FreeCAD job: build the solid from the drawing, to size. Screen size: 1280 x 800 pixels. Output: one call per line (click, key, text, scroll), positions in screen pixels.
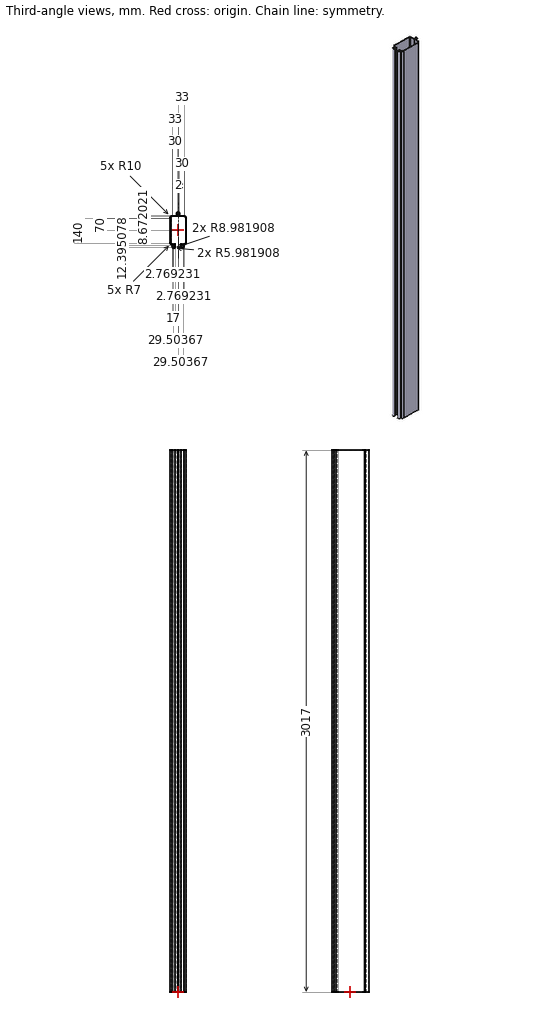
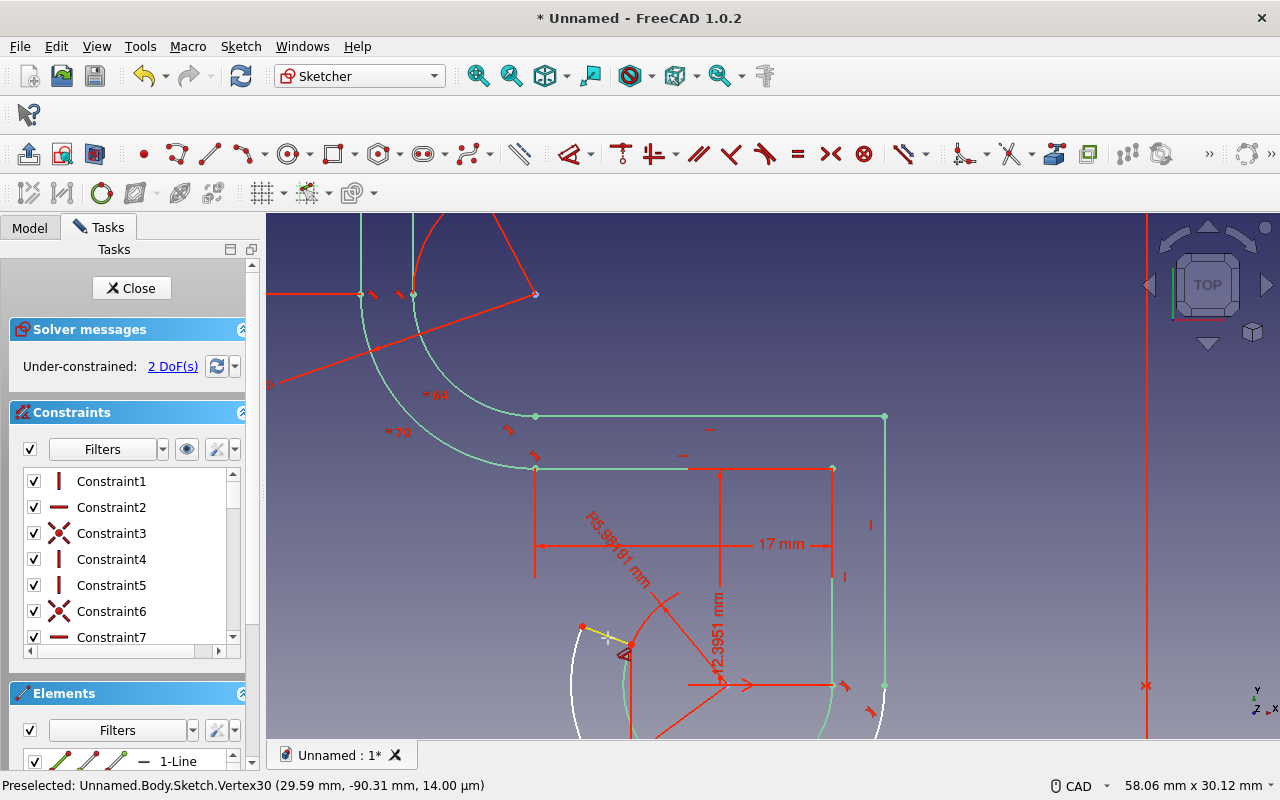
click(607, 636)
click(607, 679)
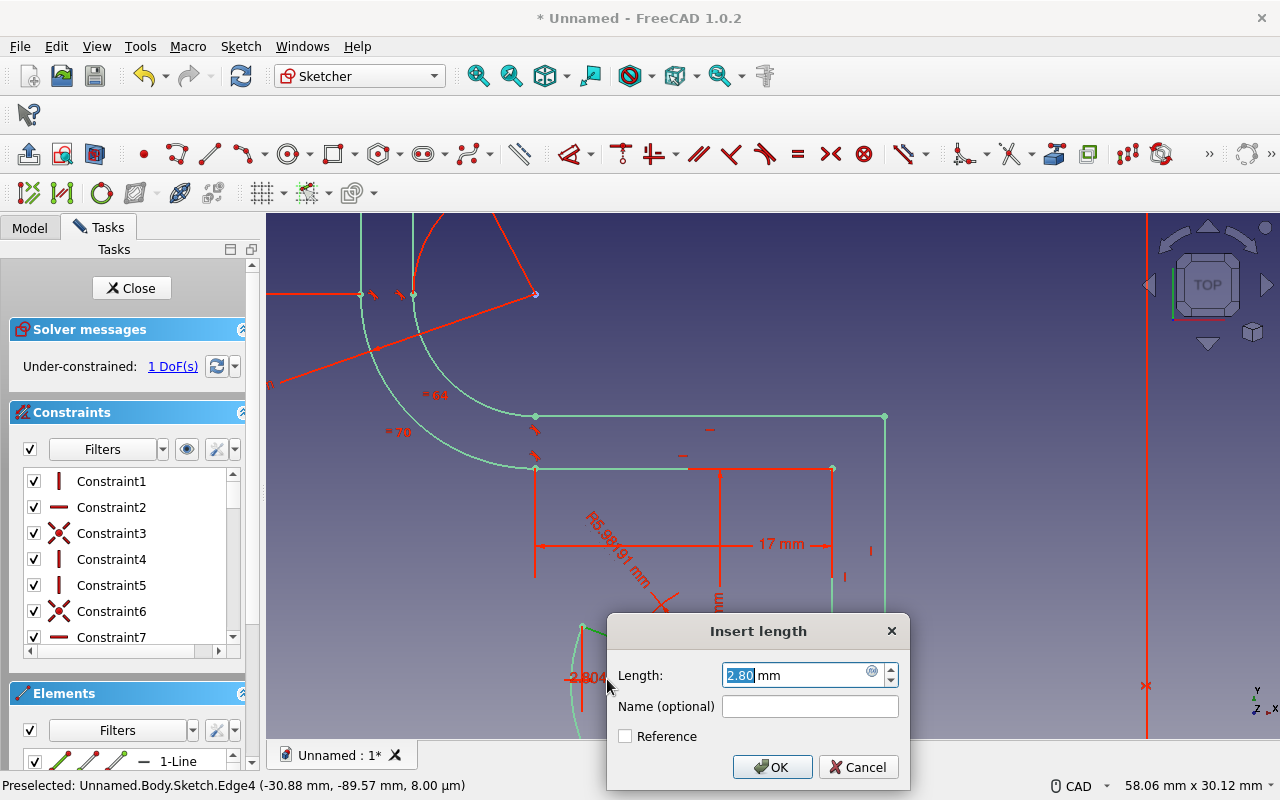
text(2.769231)
key(Return)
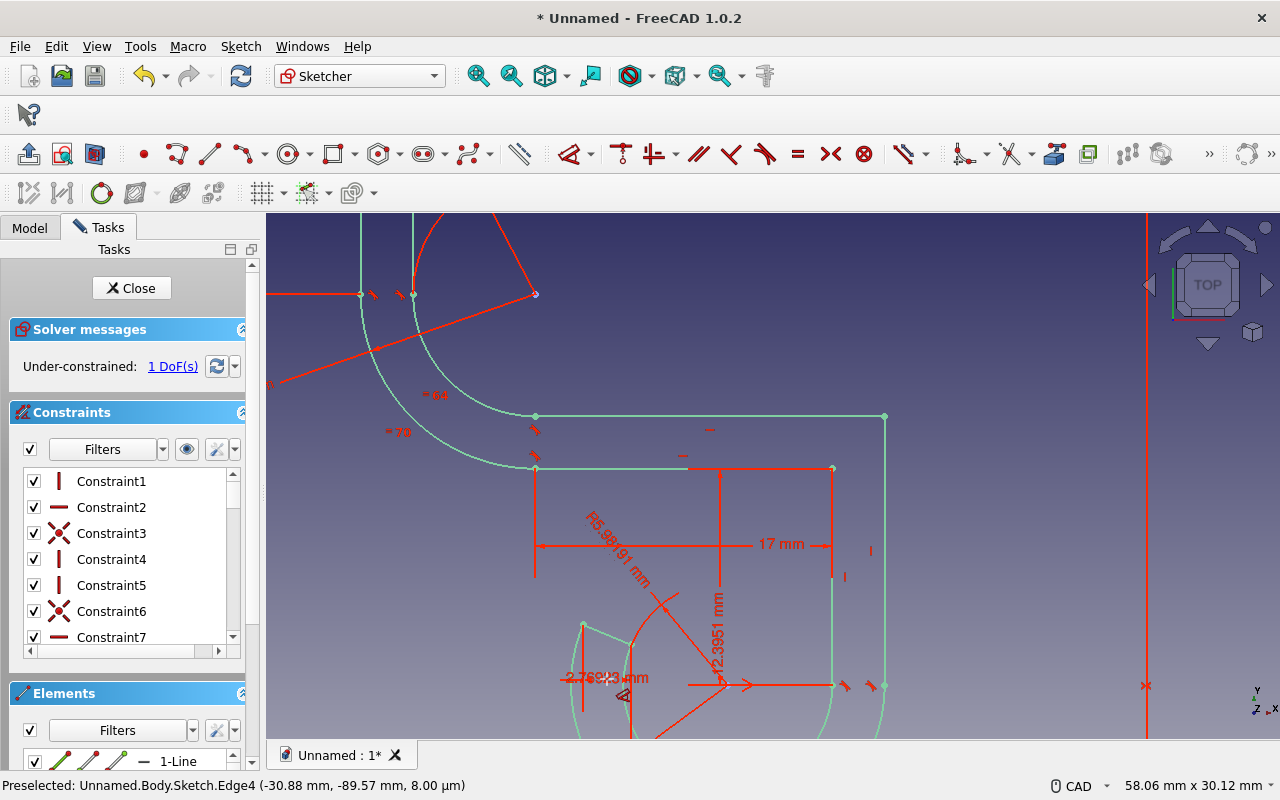
scroll(660, 617, down, 12)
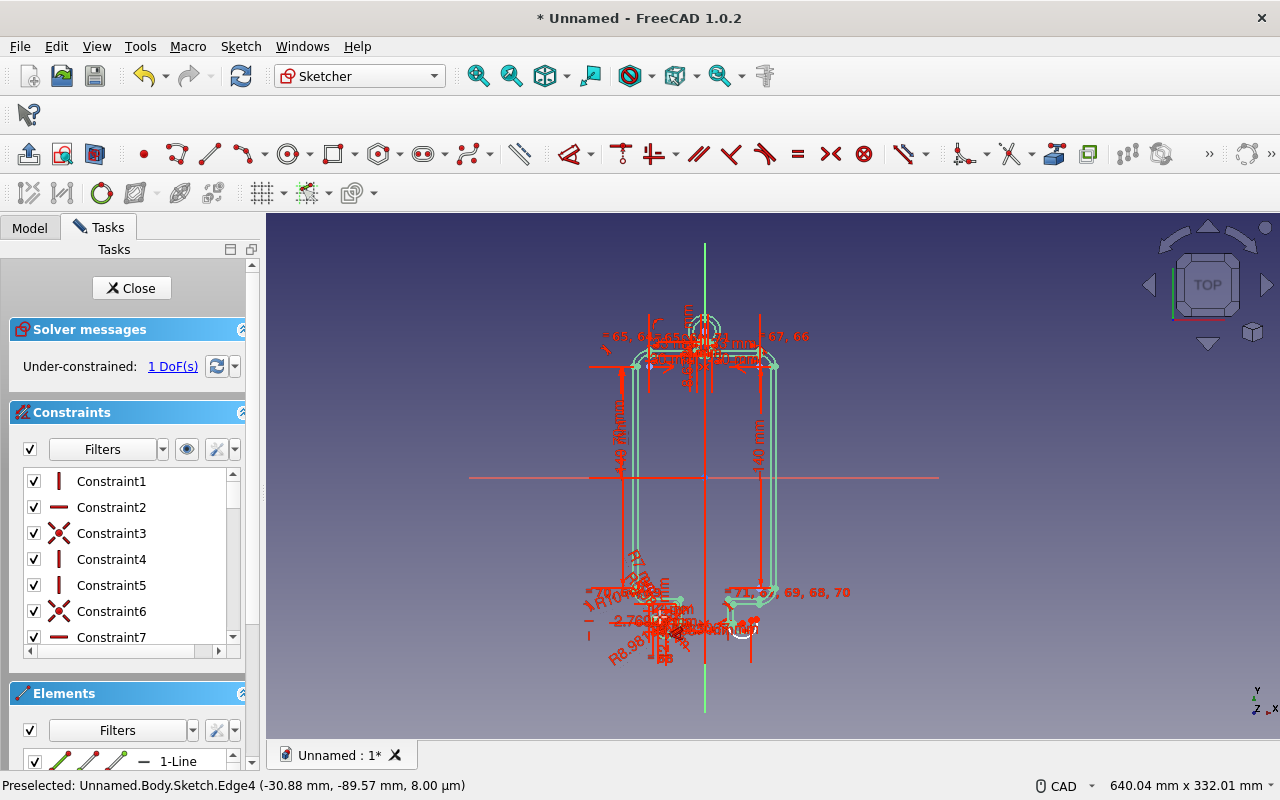
scroll(755, 620, up, 12)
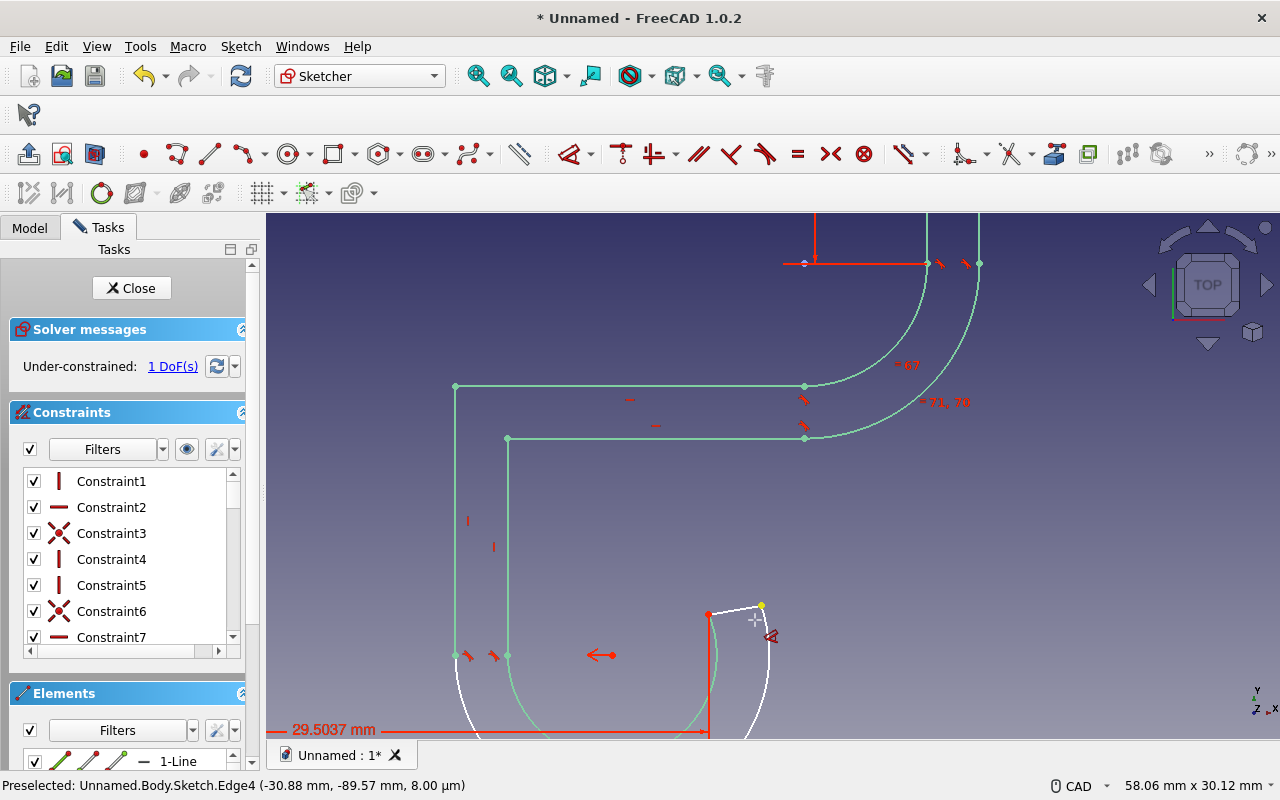
click(746, 609)
click(735, 649)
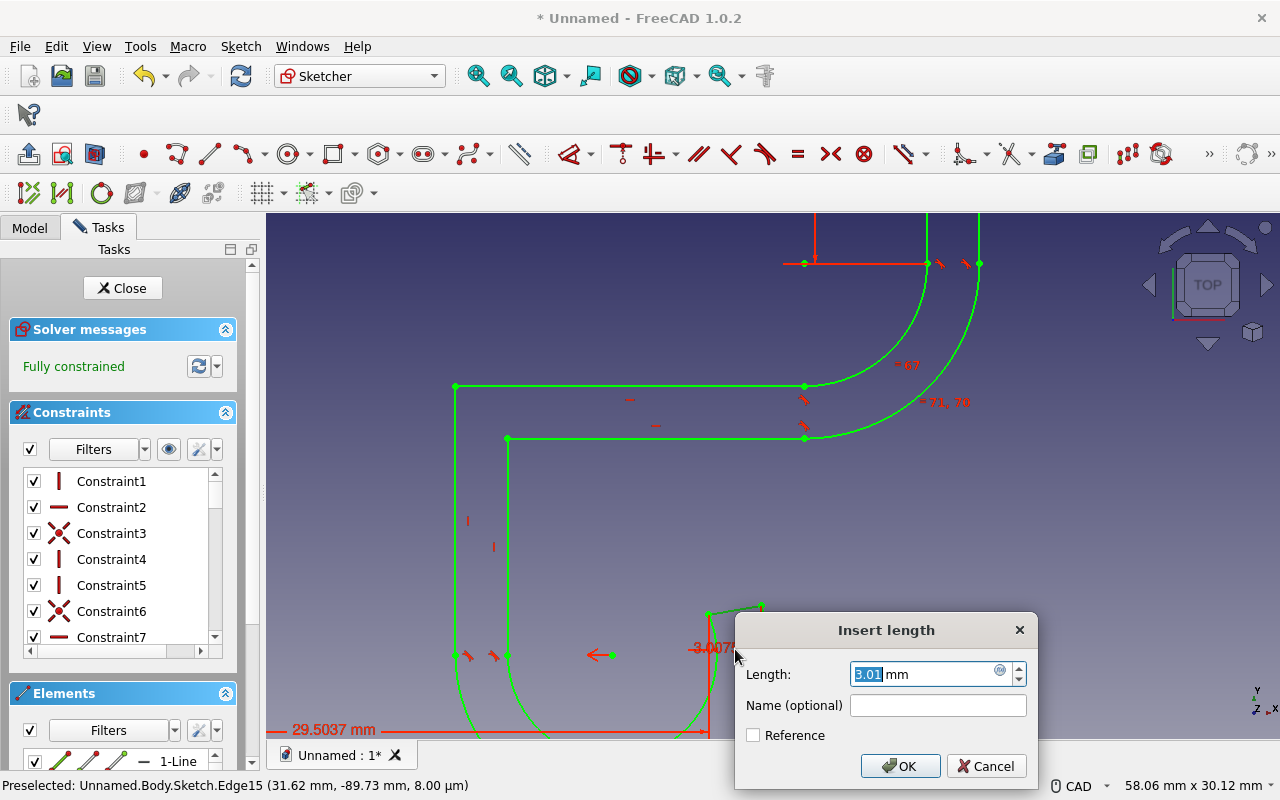
text(2.769231)
key(Return)
key(Escape)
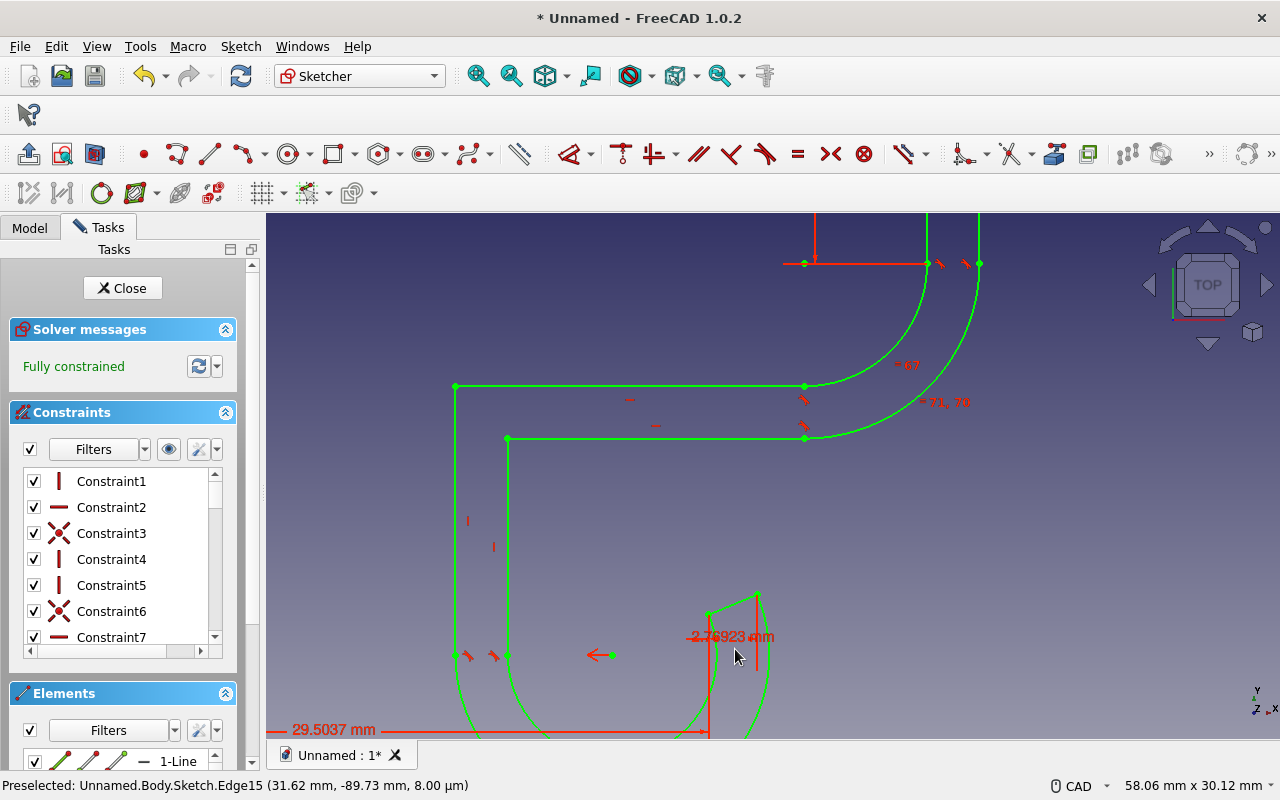
click(123, 288)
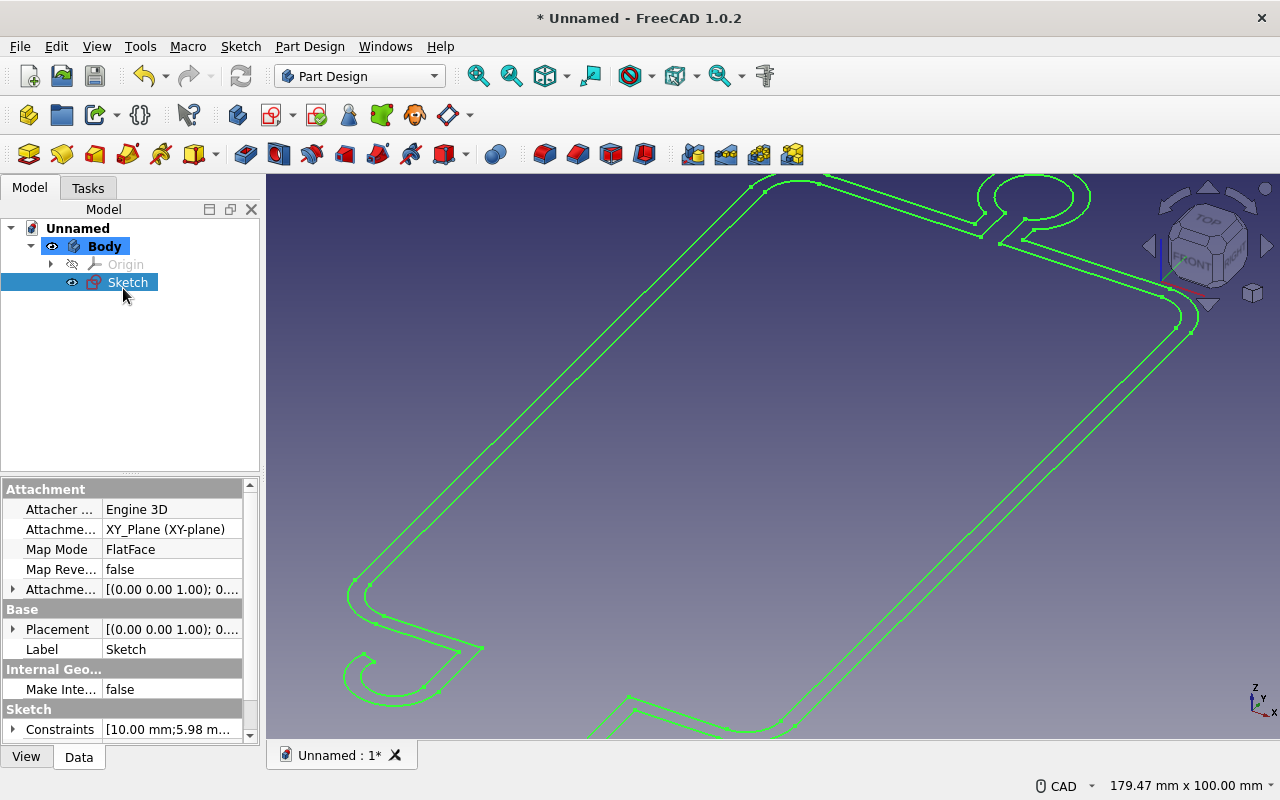
click(29, 154)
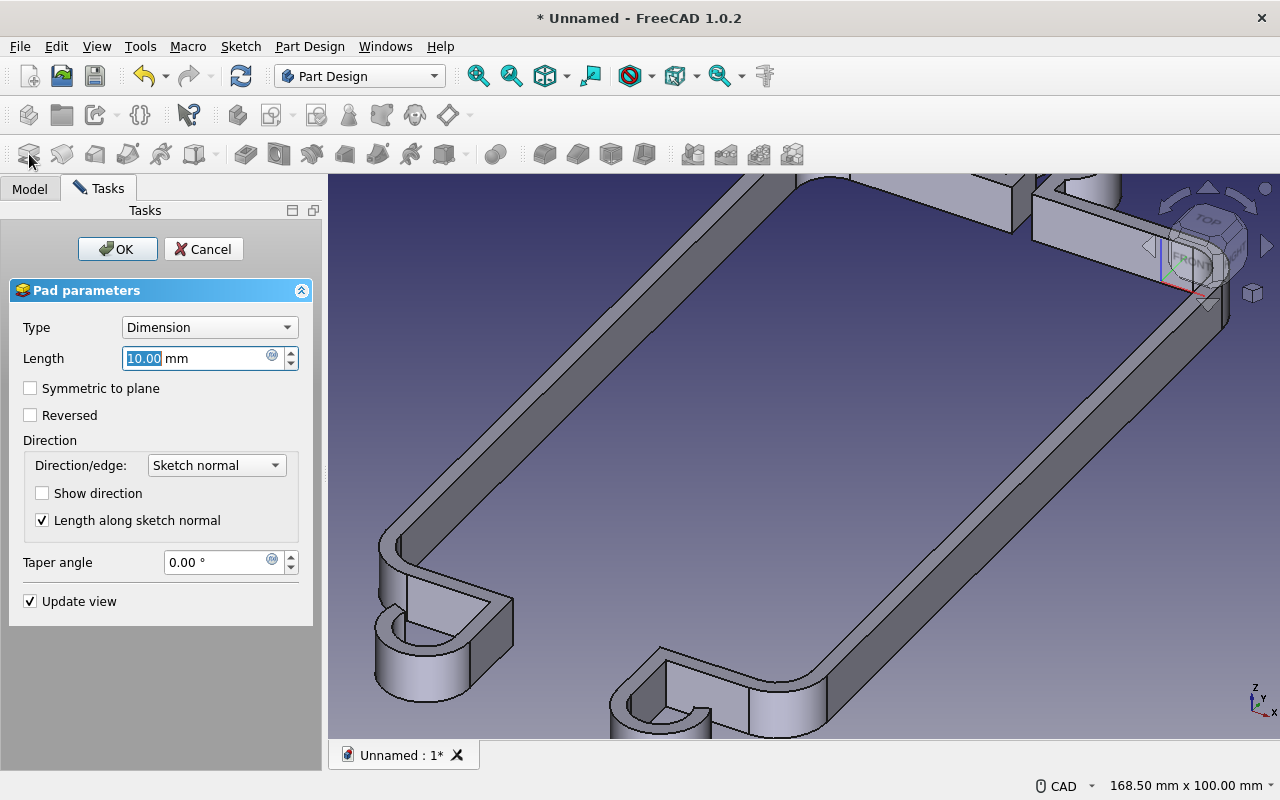
text(3017)
key(Tab)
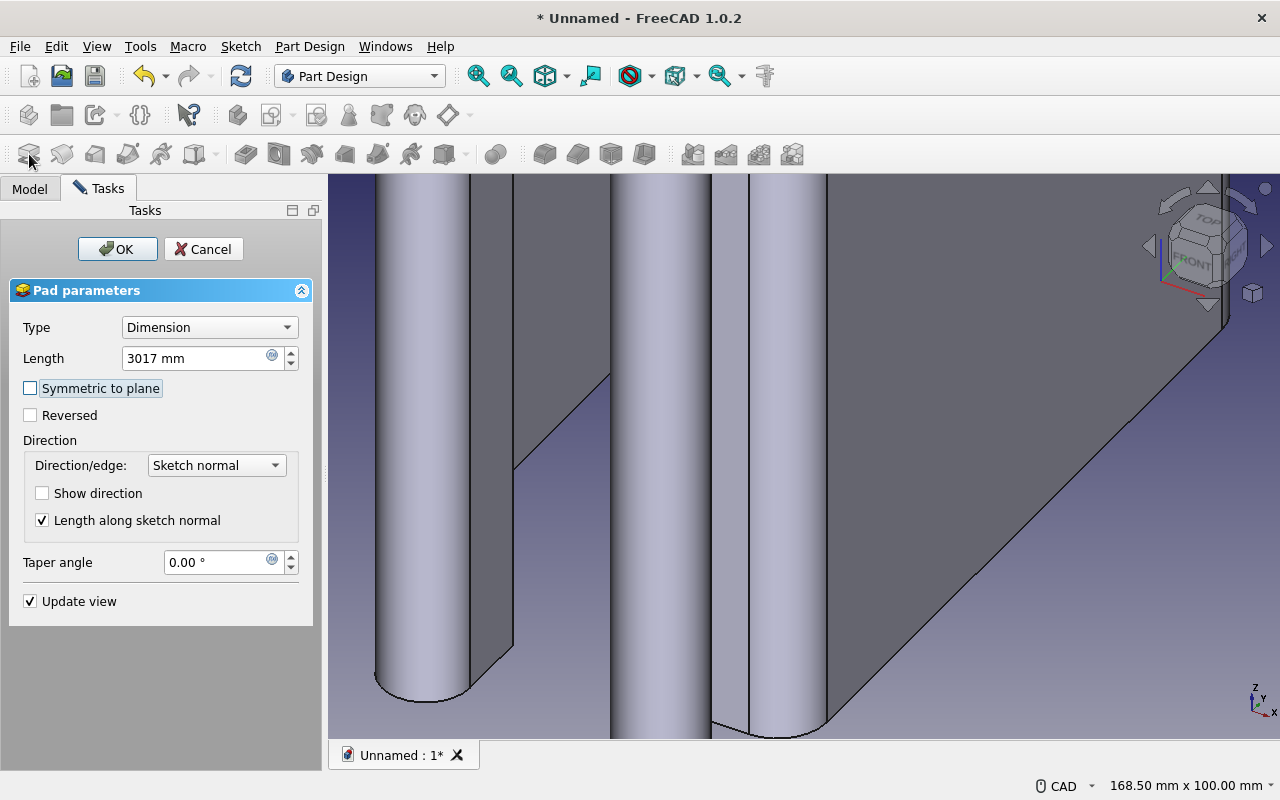
click(118, 249)